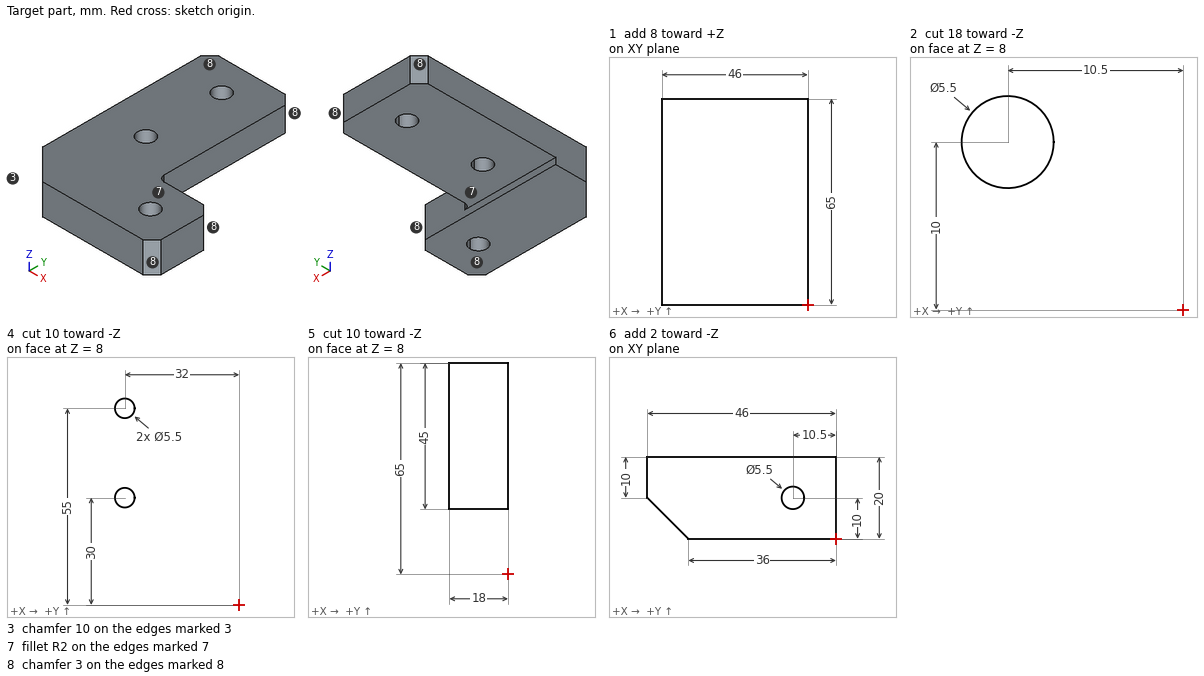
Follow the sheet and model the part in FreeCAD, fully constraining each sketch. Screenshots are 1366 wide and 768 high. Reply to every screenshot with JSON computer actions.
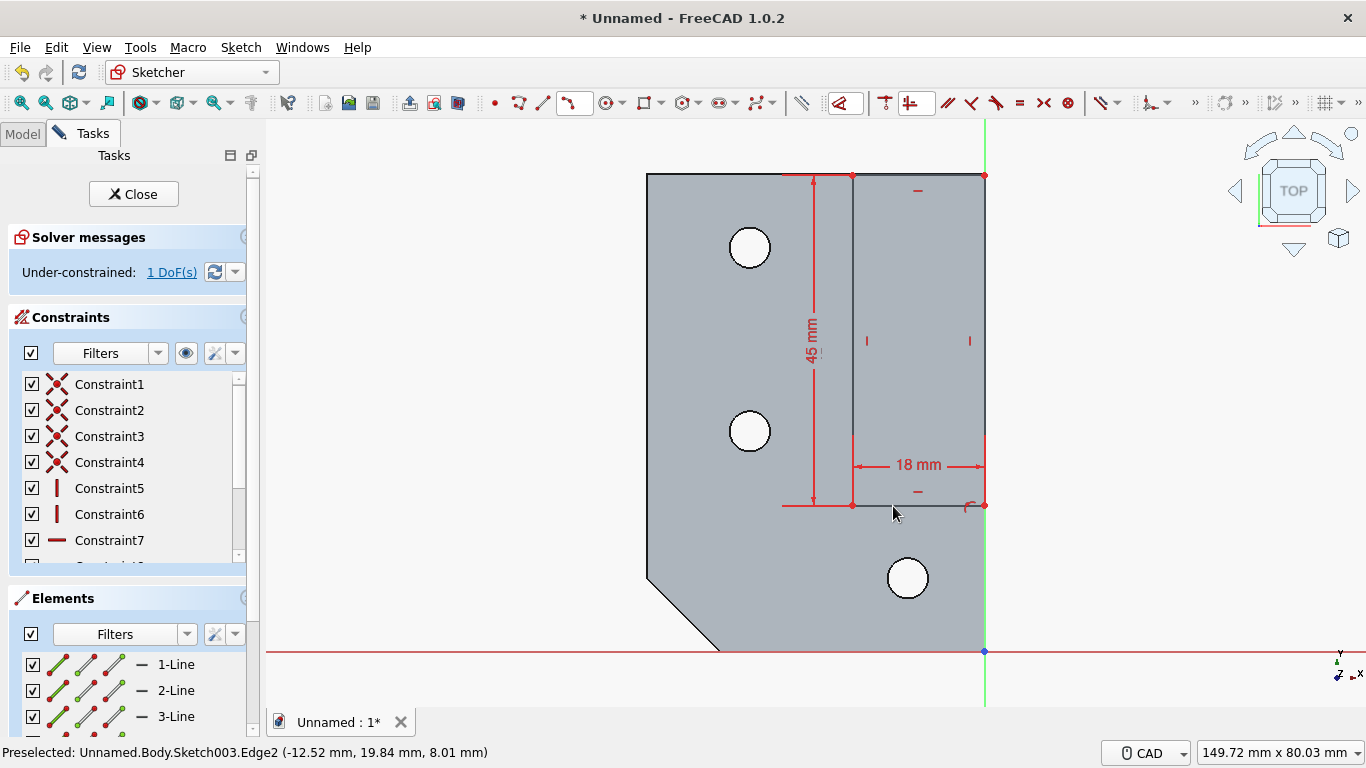
{"action": "left_click", "coordinate": [853, 175]}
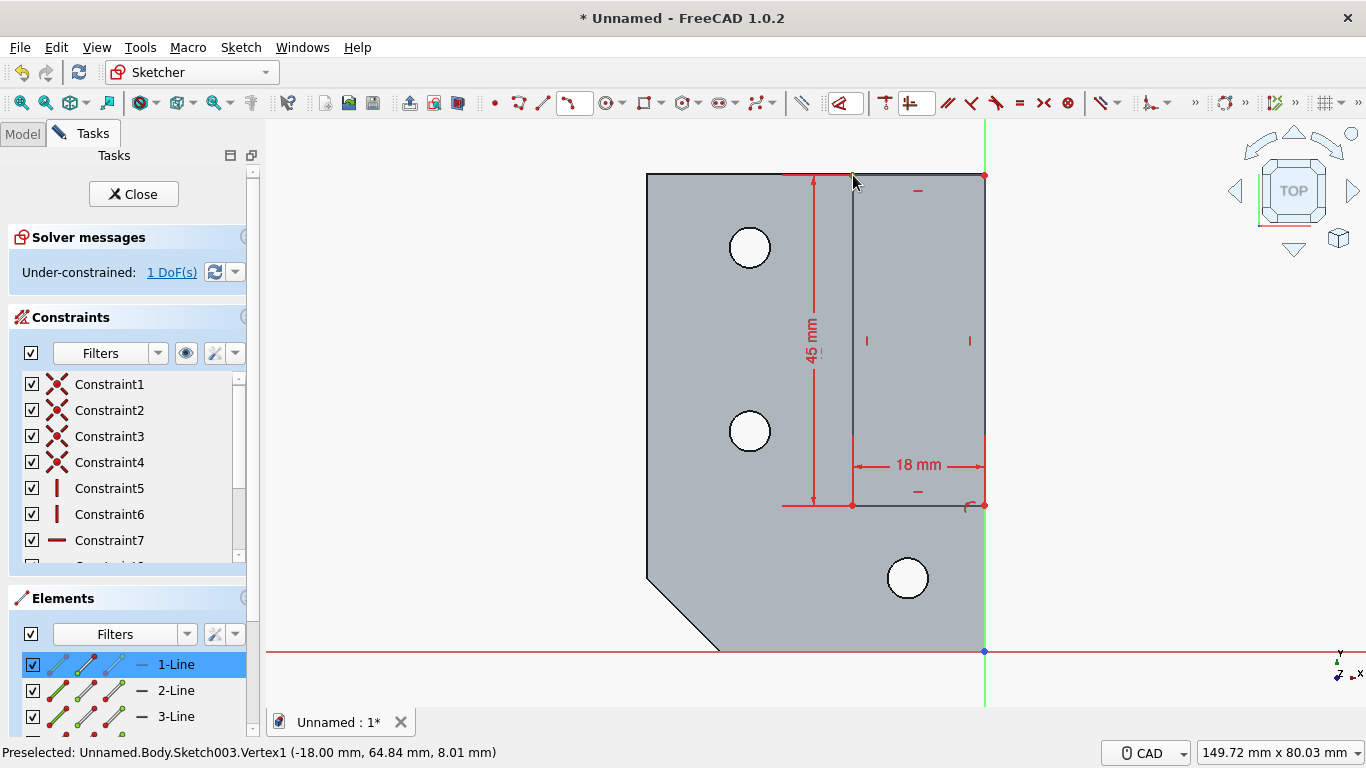
{"action": "key", "text": "i"}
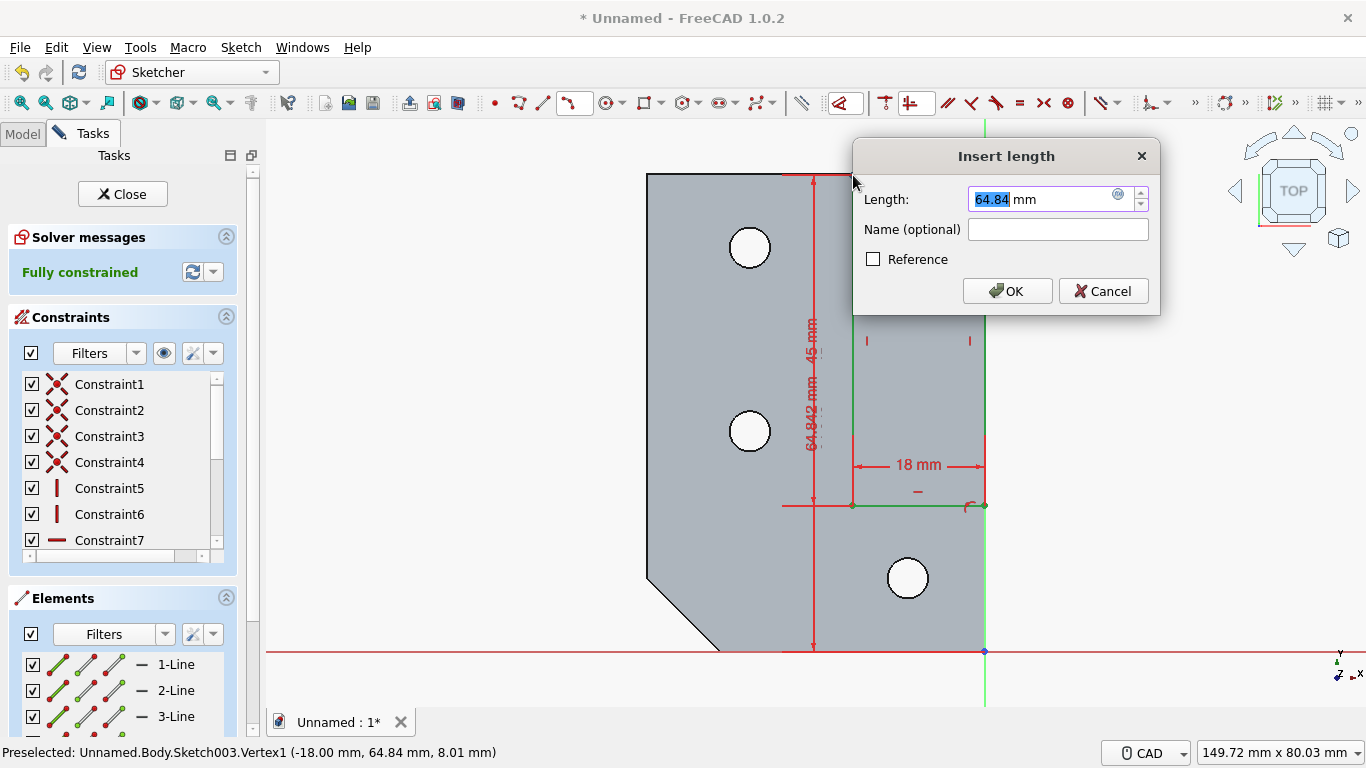
{"action": "type", "text": "65"}
{"action": "key", "text": "Return"}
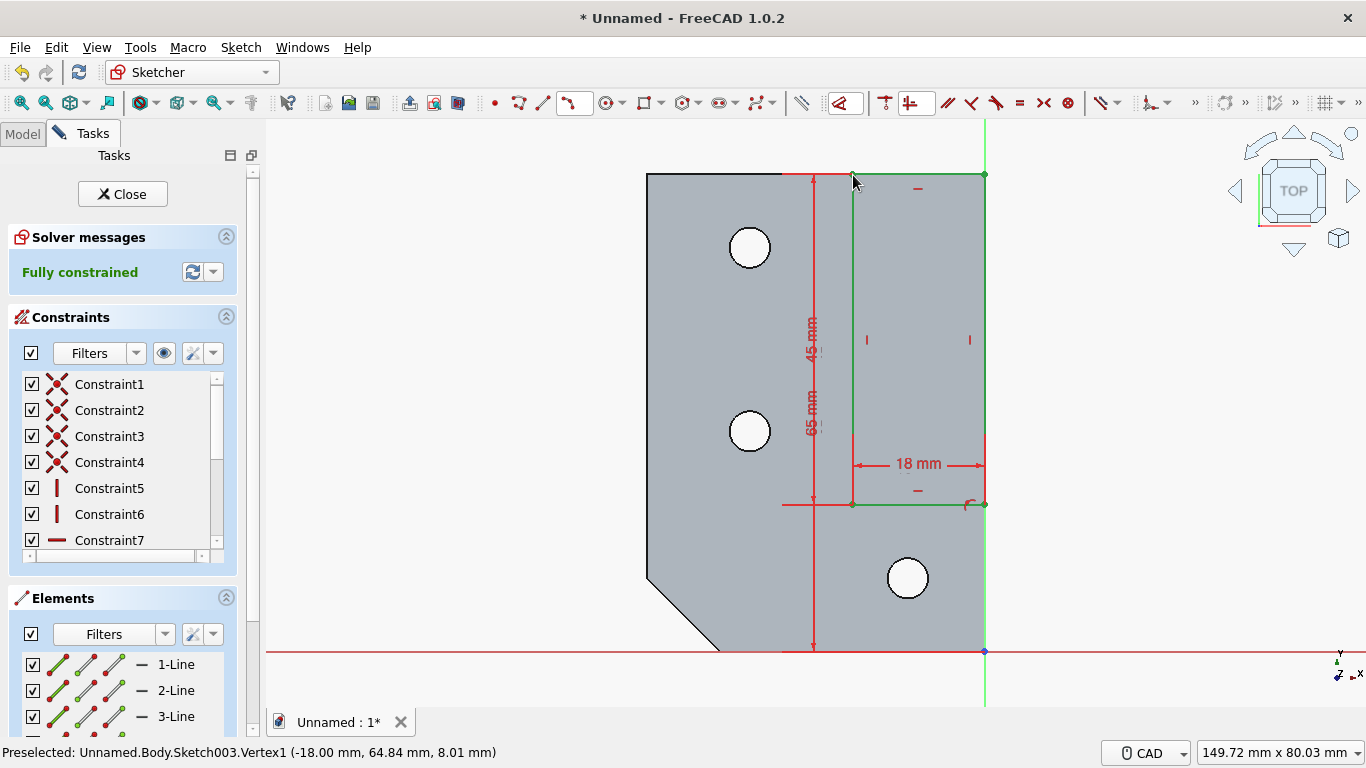
{"action": "left_click", "coordinate": [123, 194]}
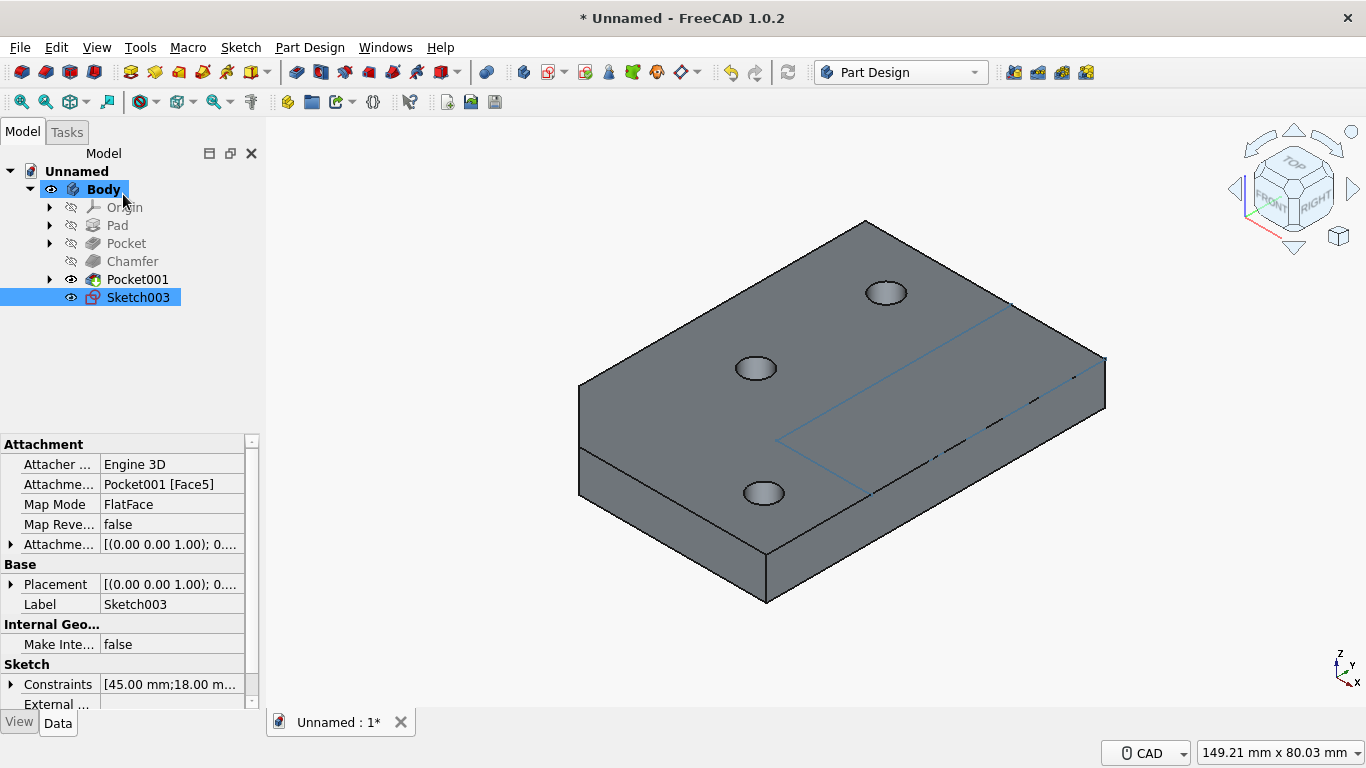
{"action": "left_click", "coordinate": [298, 72]}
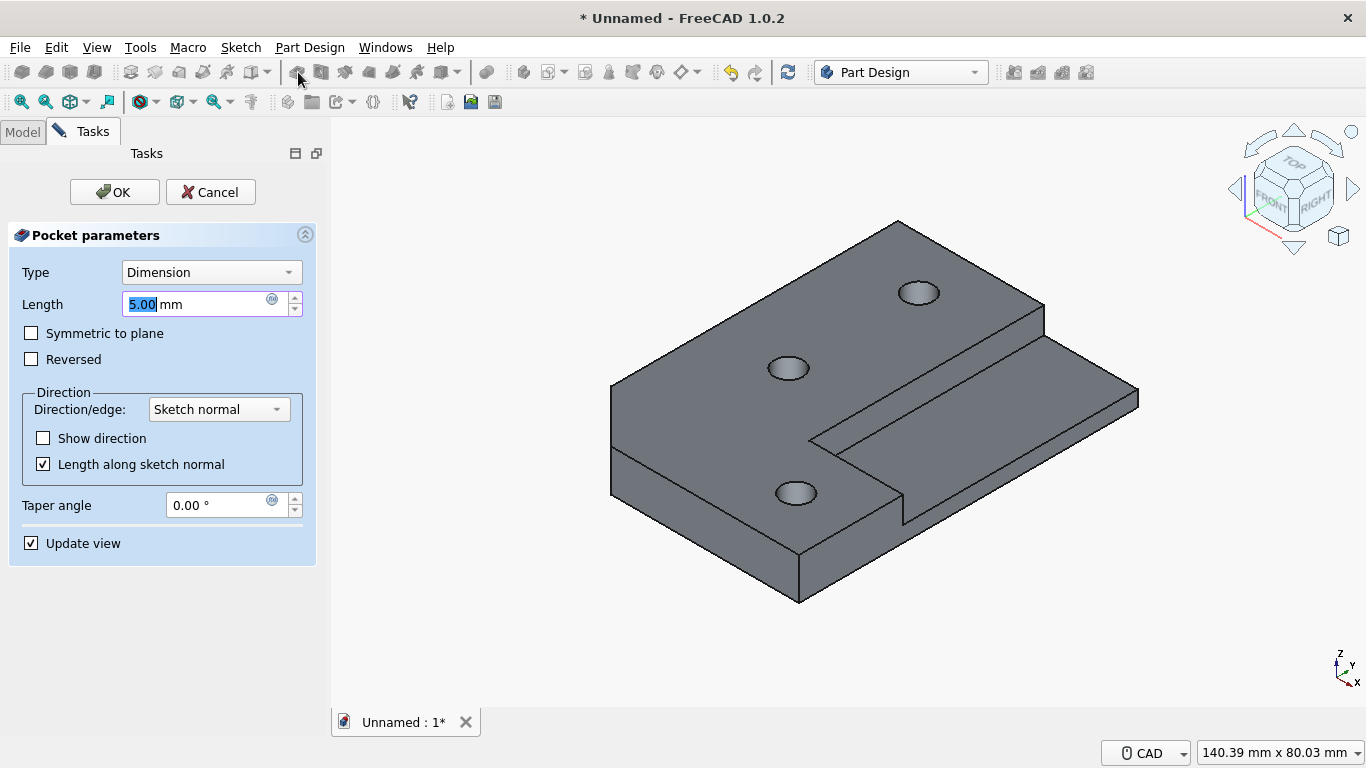
{"action": "type", "text": "10"}
{"action": "key", "text": "Tab"}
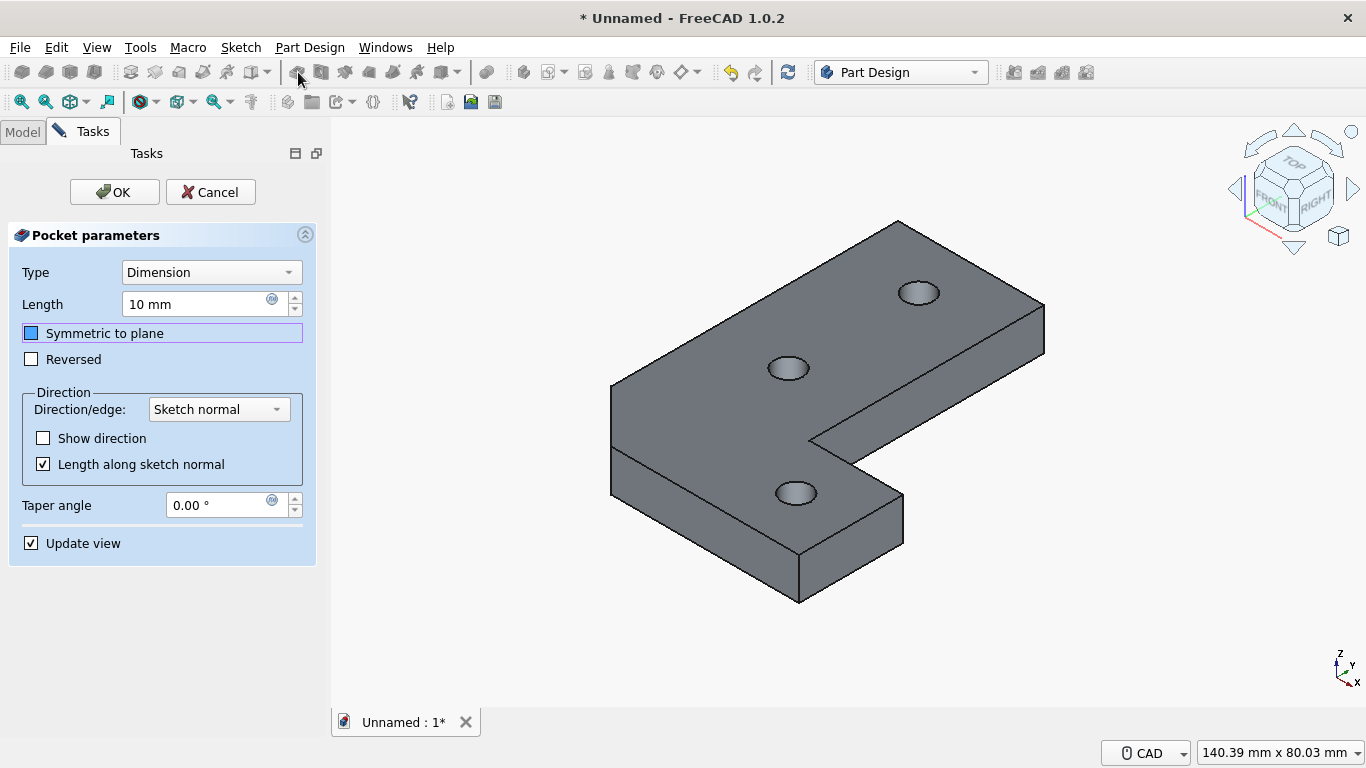
{"action": "left_click", "coordinate": [115, 192]}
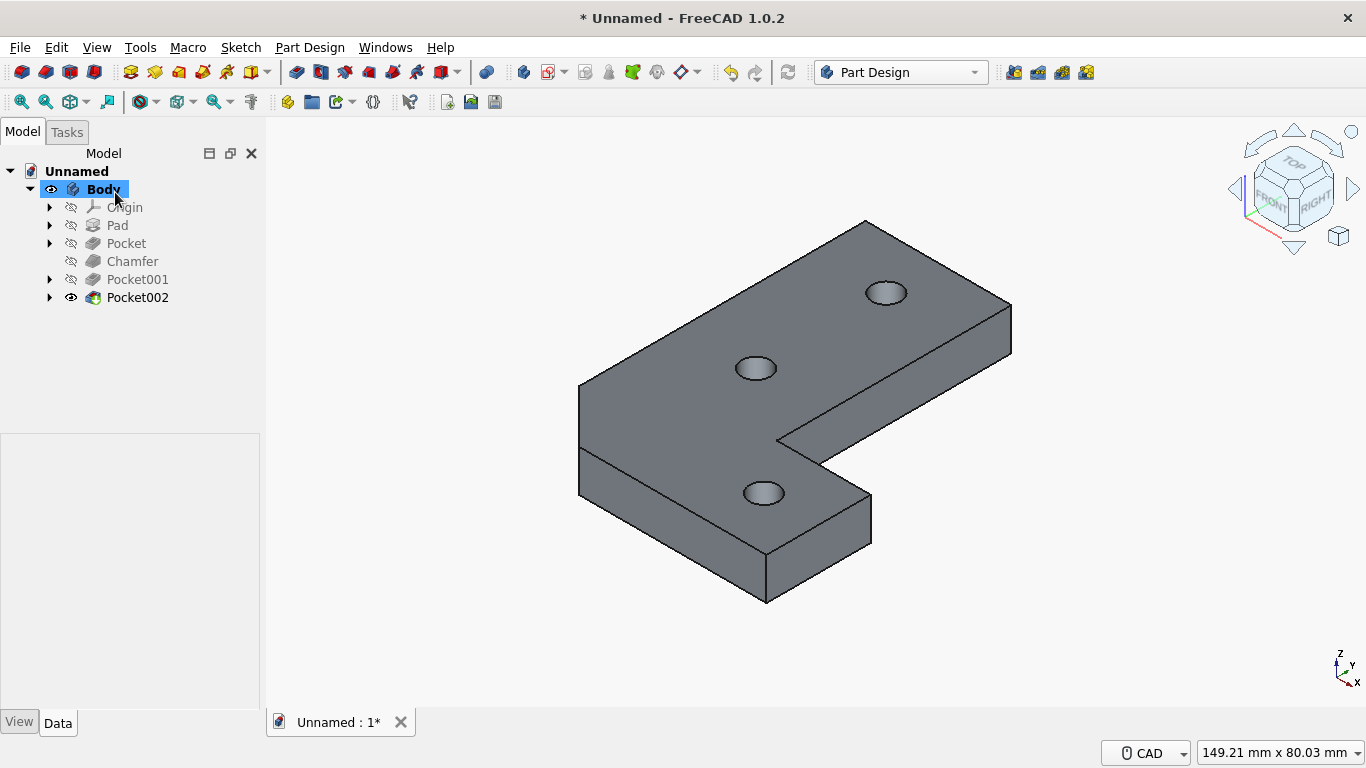
{"action": "left_click", "coordinate": [548, 72]}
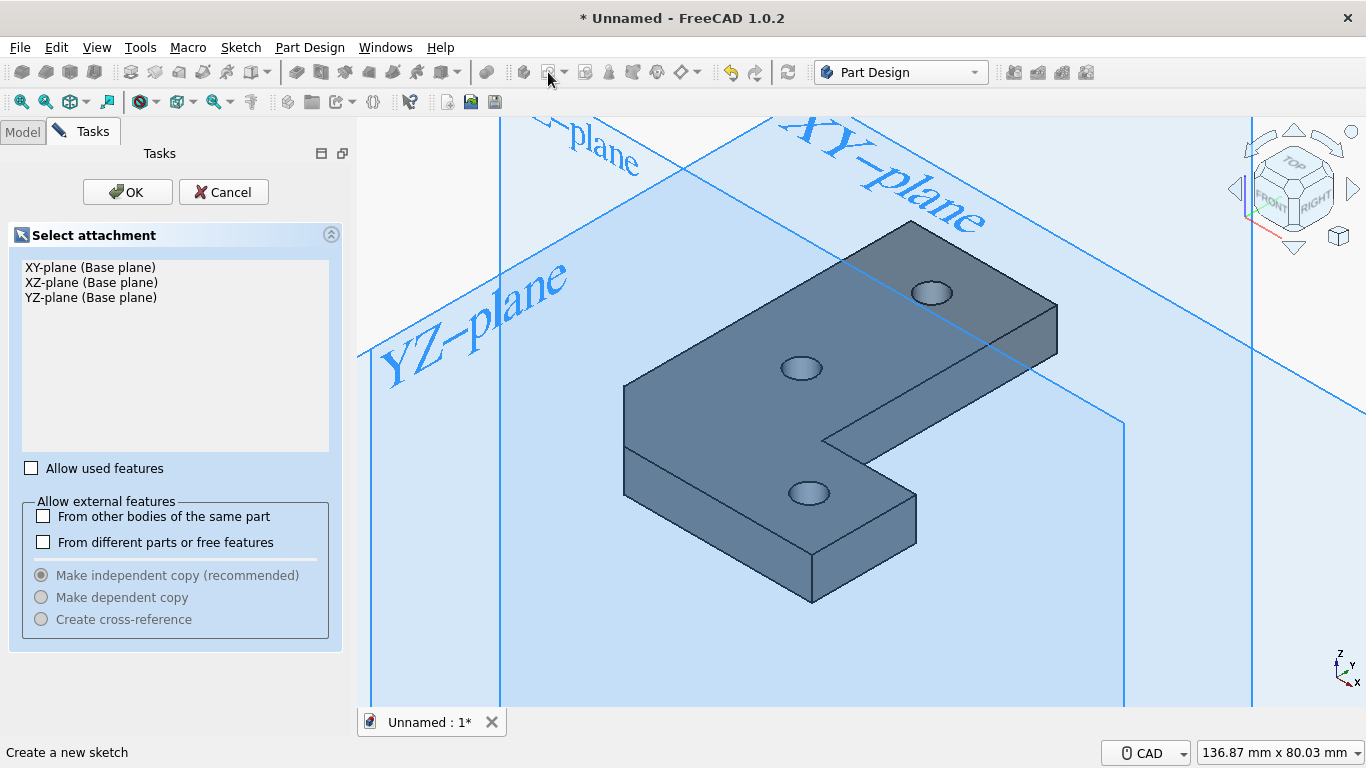
{"action": "left_click", "coordinate": [82, 268]}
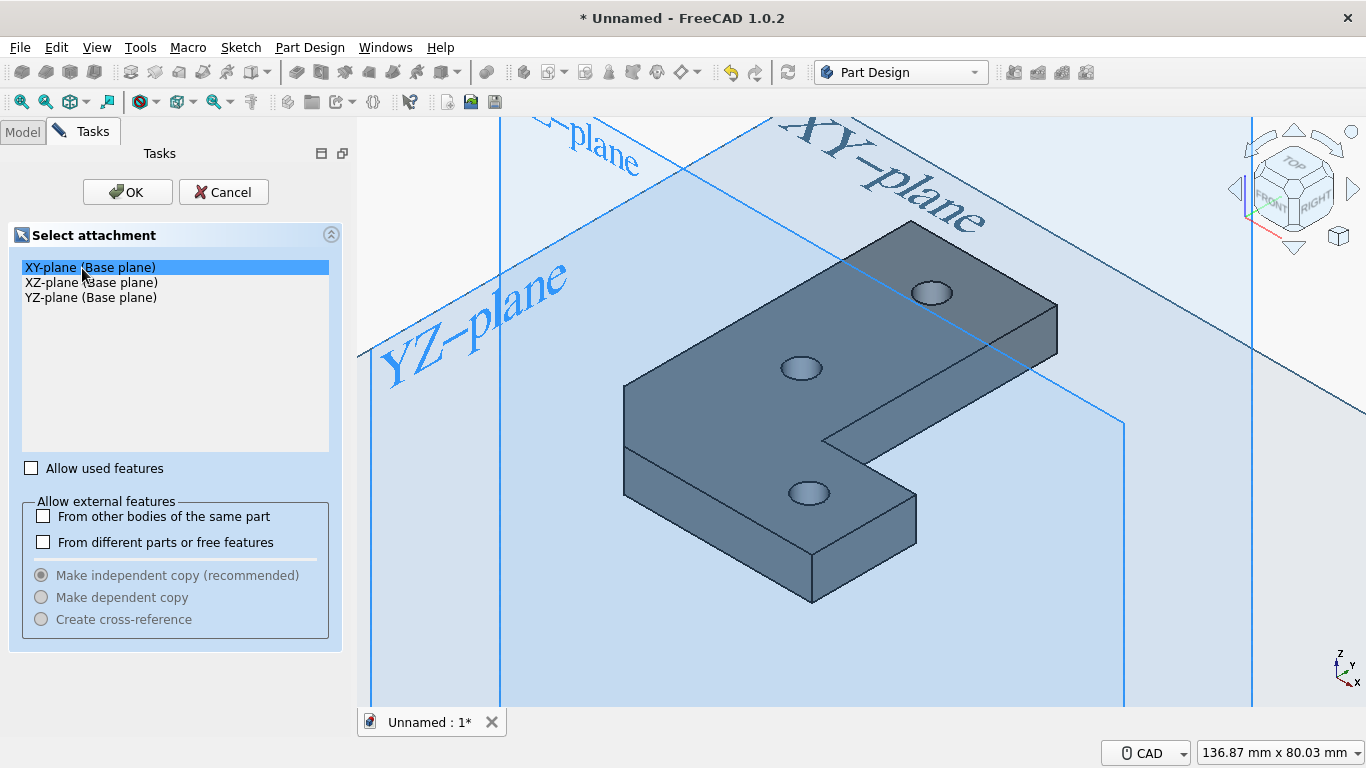
{"action": "left_click", "coordinate": [128, 192]}